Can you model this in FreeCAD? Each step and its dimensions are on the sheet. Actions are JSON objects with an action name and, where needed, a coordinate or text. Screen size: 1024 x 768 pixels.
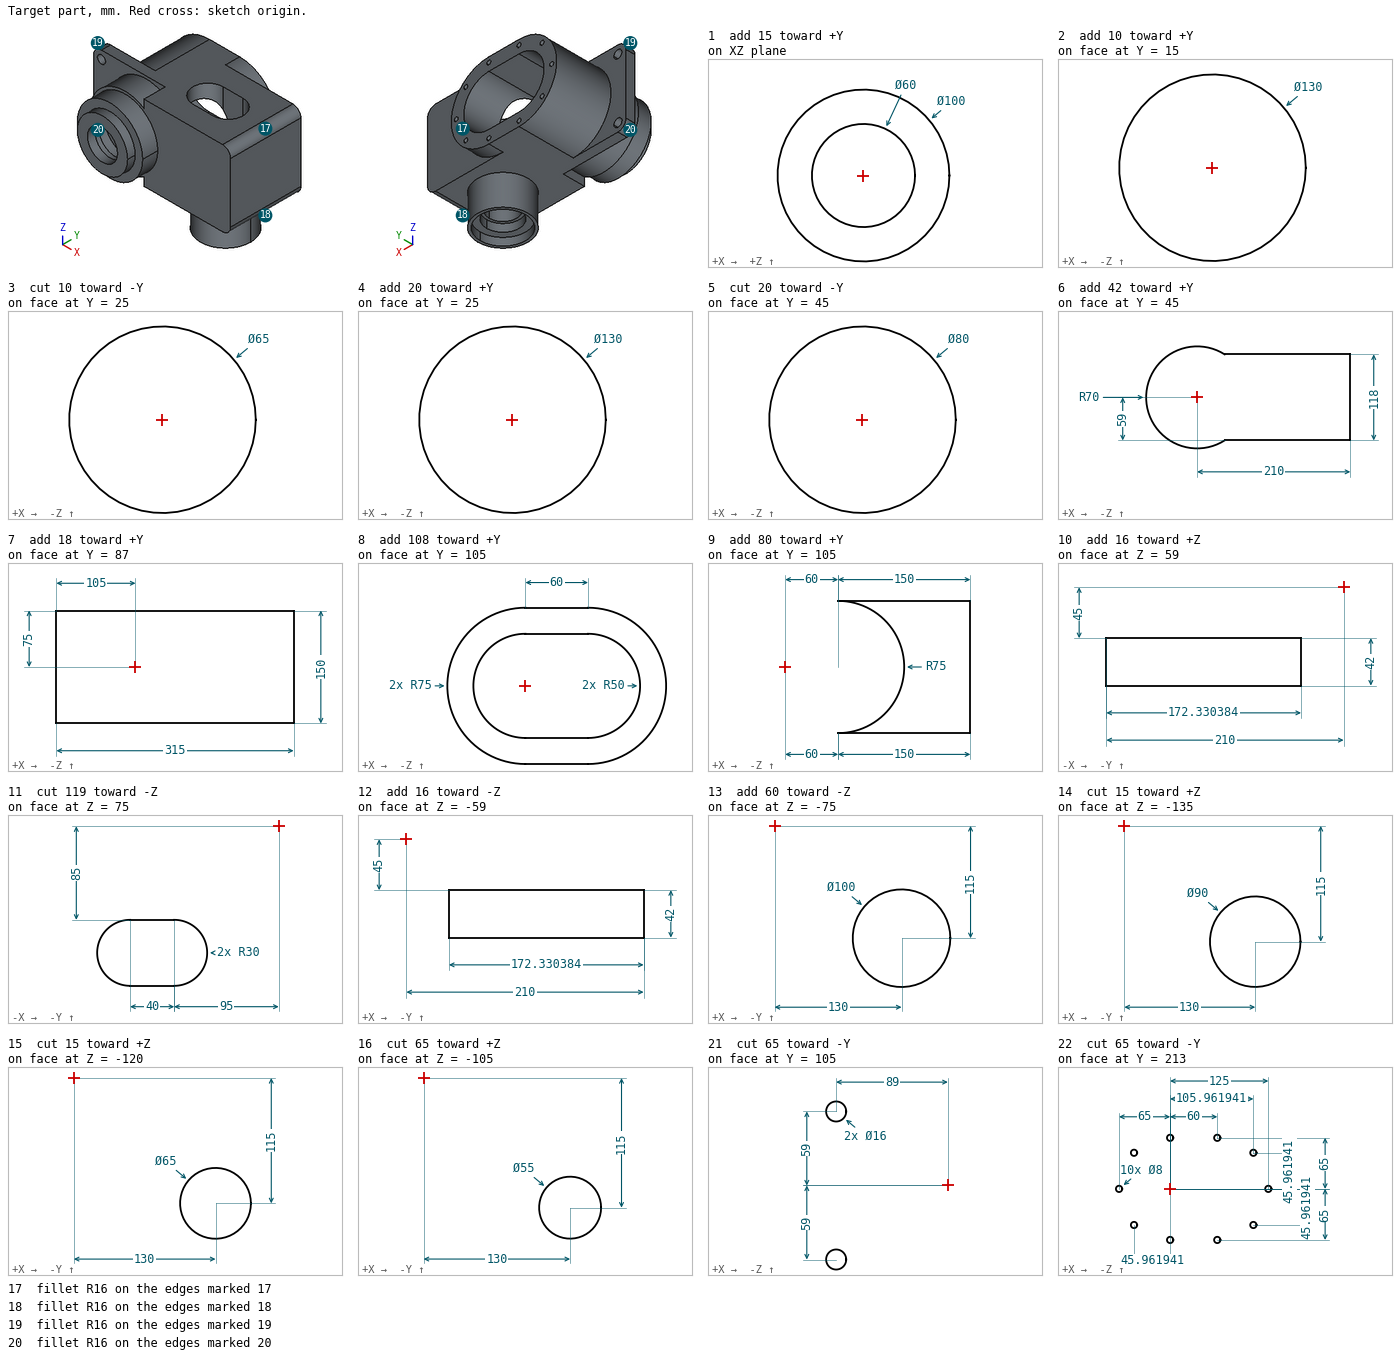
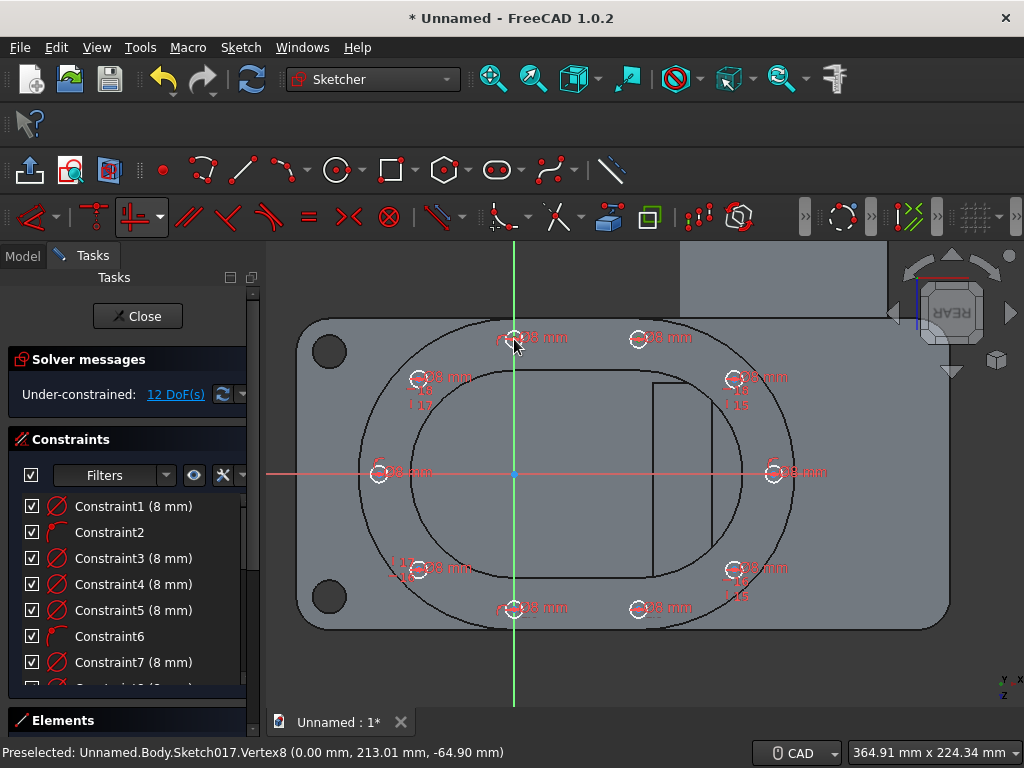
{"action": "key", "text": "h"}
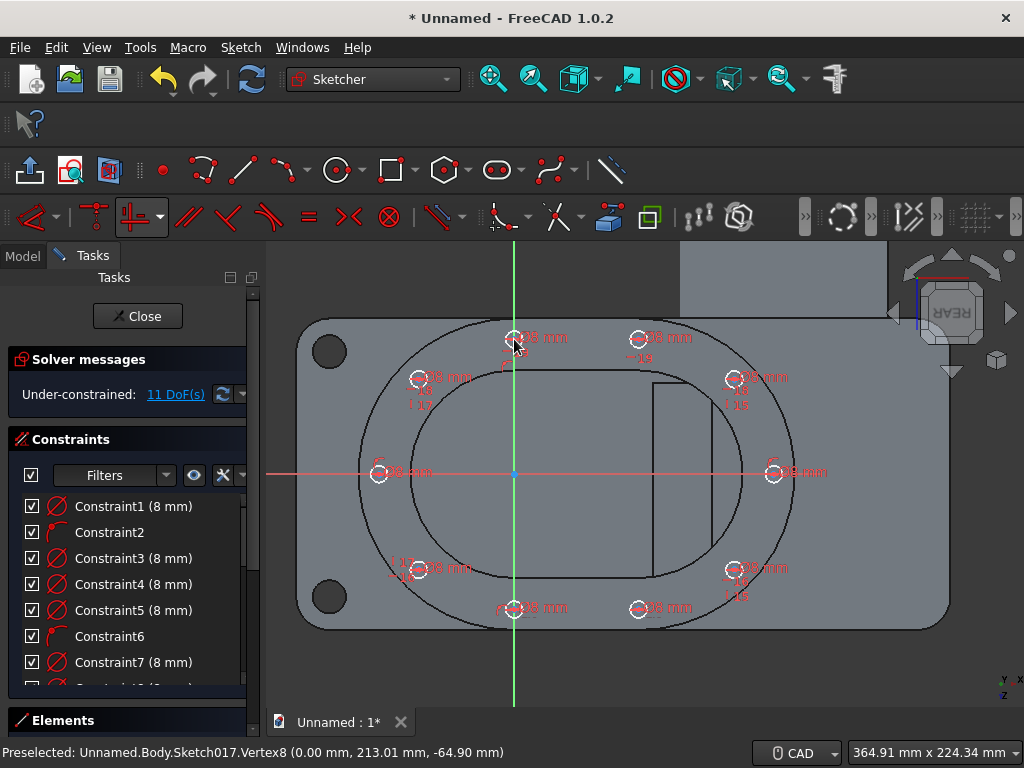
{"action": "left_click", "coordinate": [639, 339]}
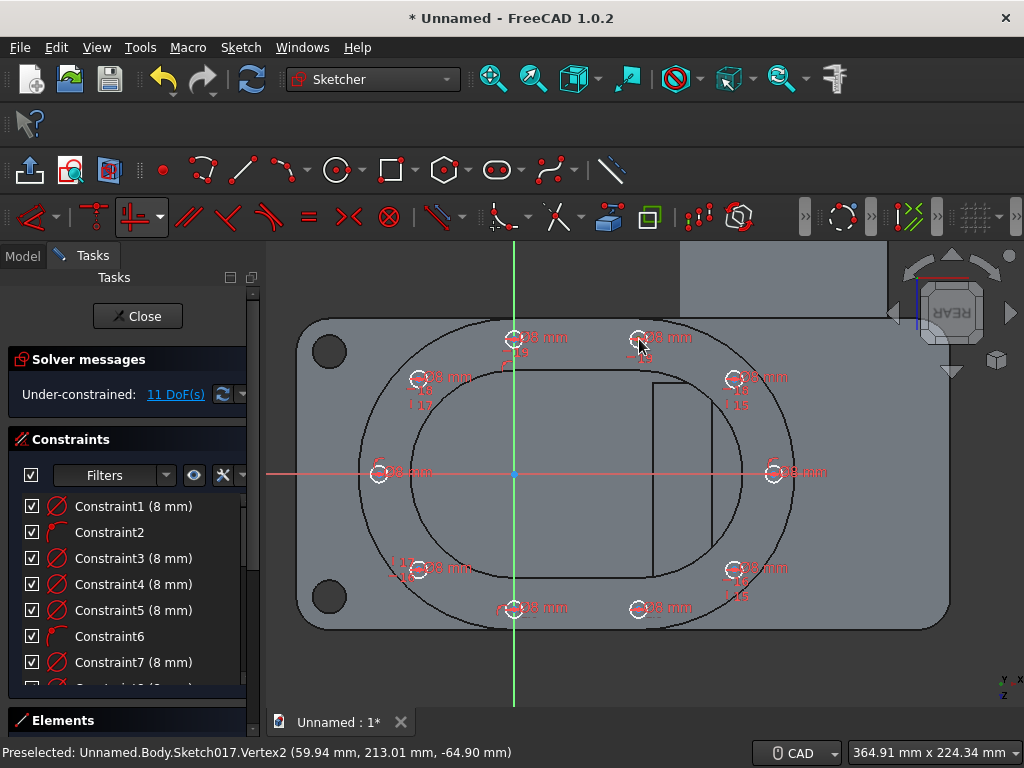
{"action": "left_click", "coordinate": [639, 610]}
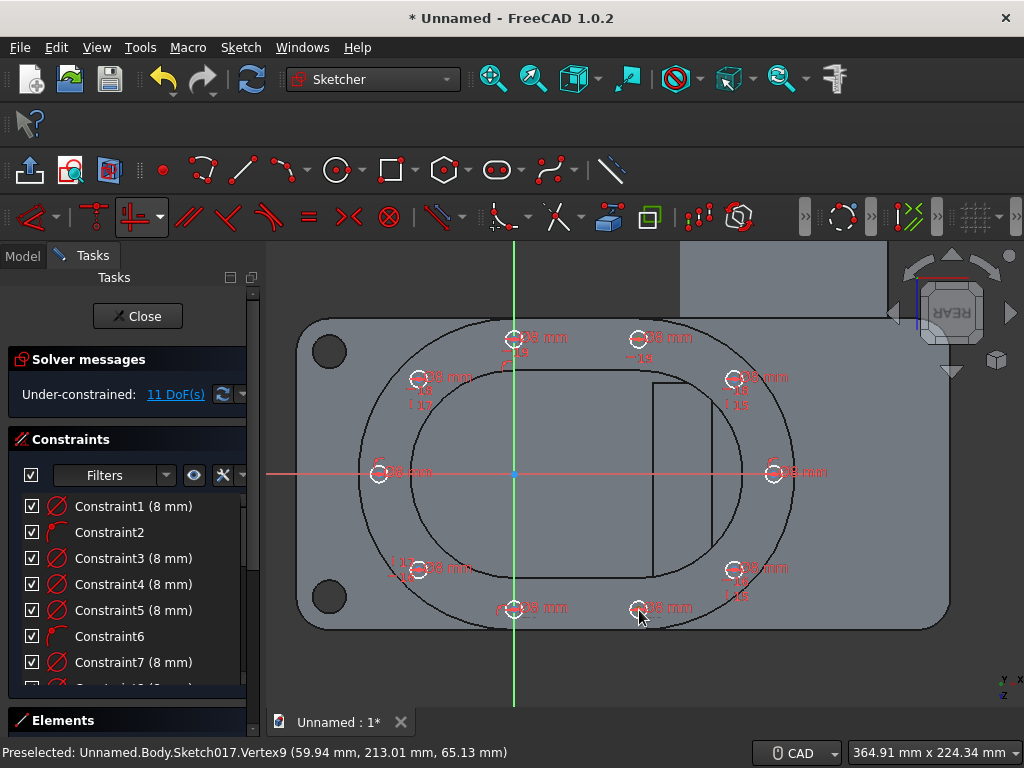
{"action": "key", "text": "v"}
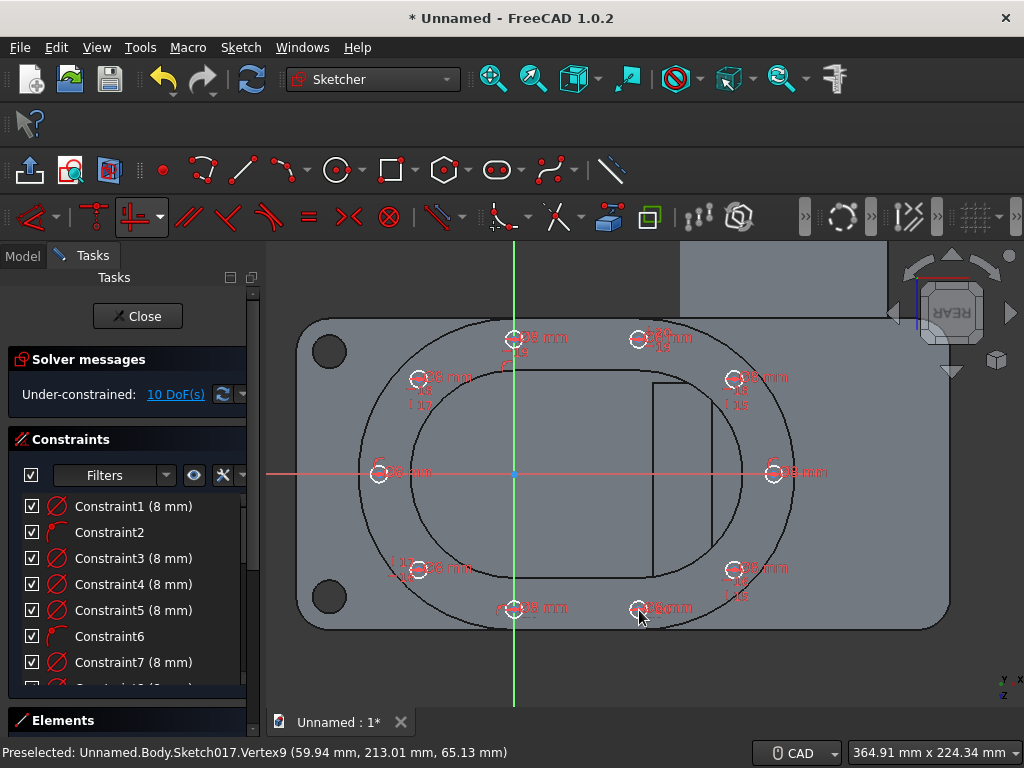
{"action": "left_click", "coordinate": [639, 610]}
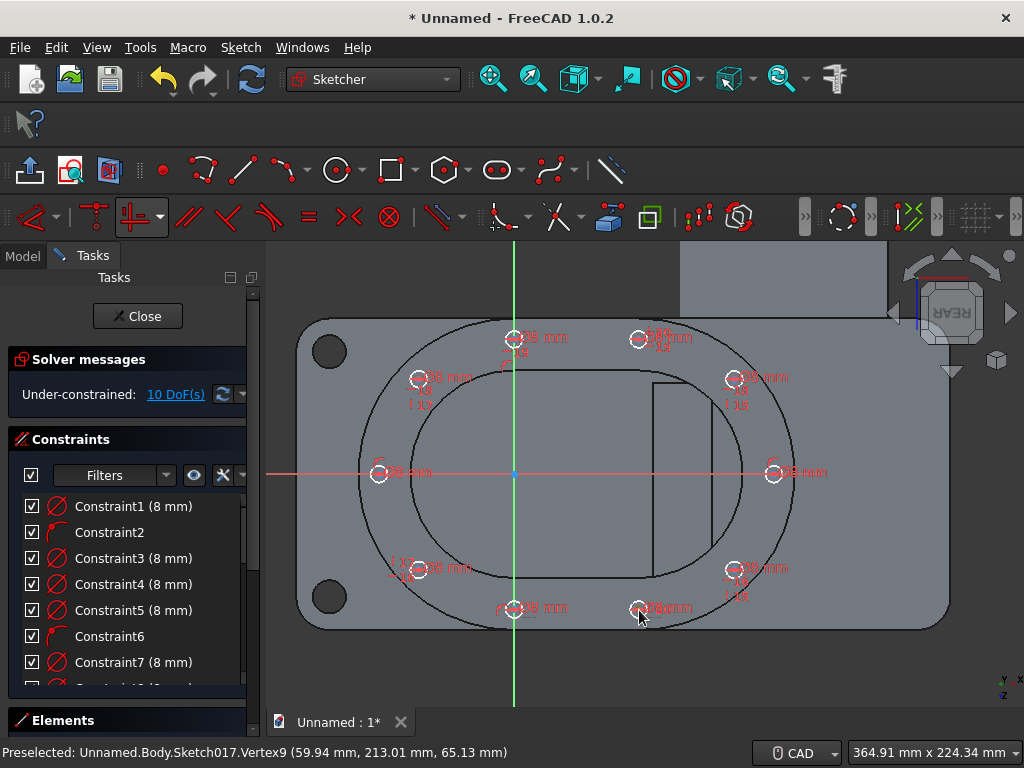
{"action": "left_click", "coordinate": [514, 610]}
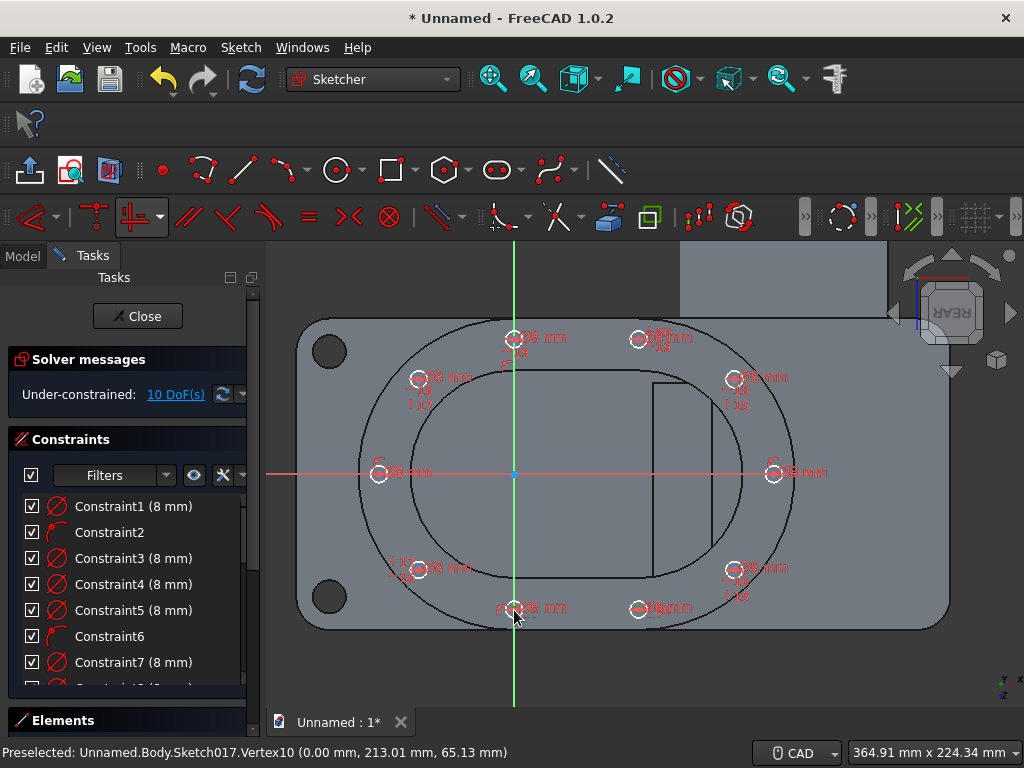
{"action": "left_click", "coordinate": [162, 218]}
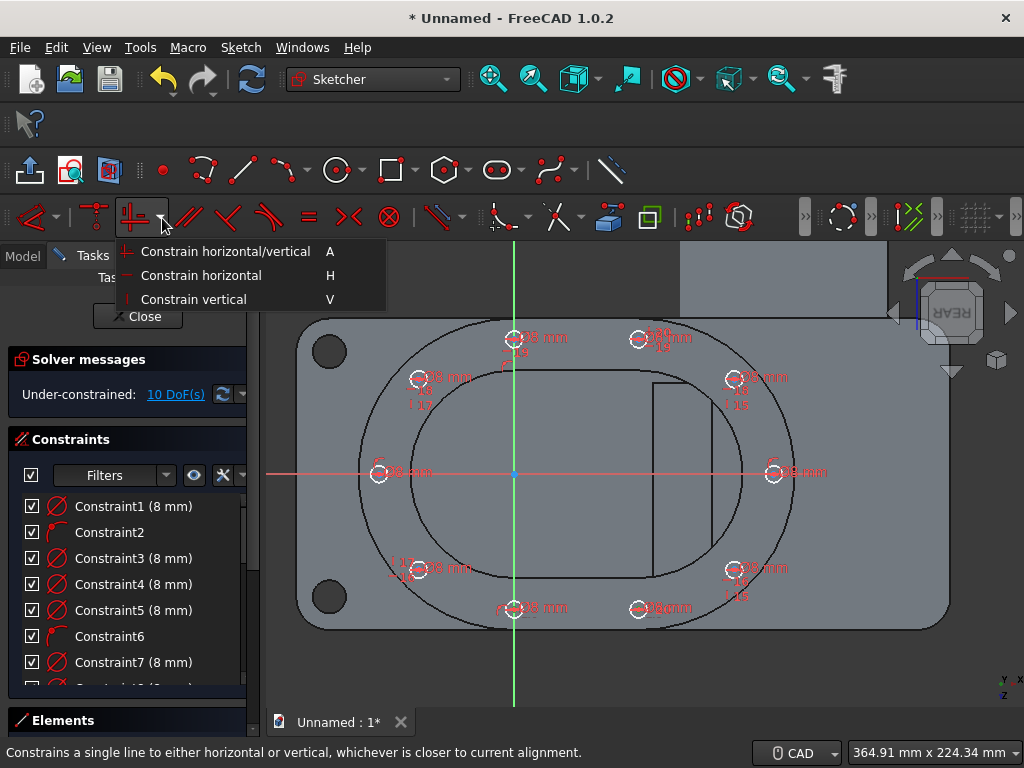
{"action": "left_click", "coordinate": [251, 275]}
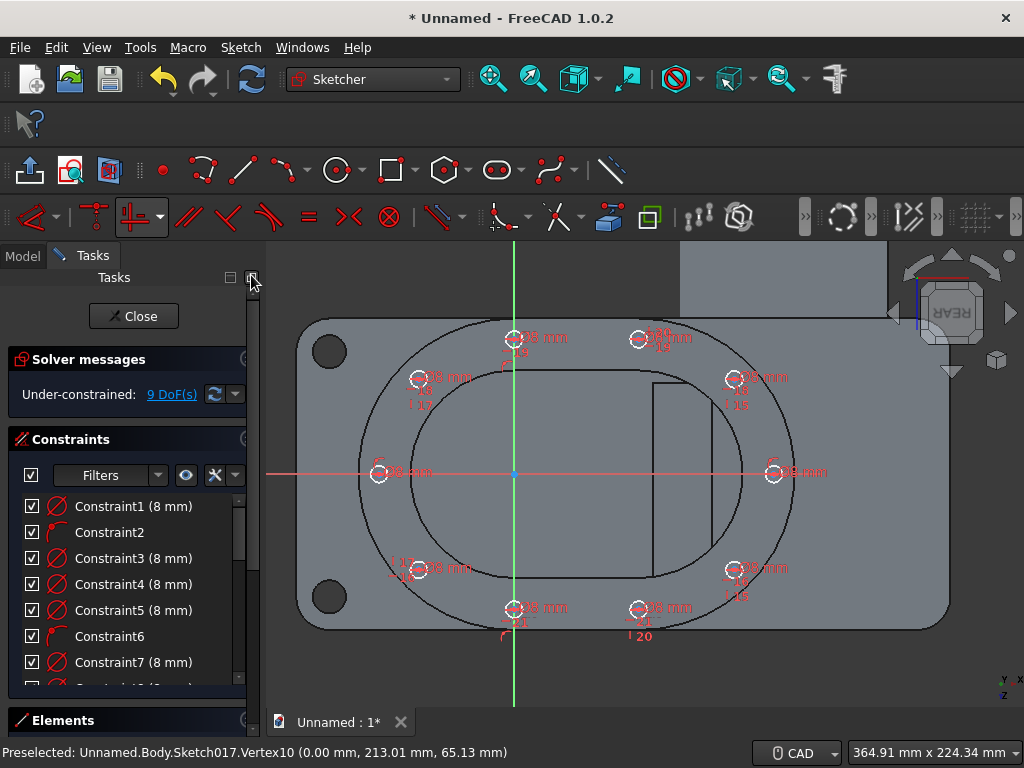
{"action": "left_click", "coordinate": [32, 218]}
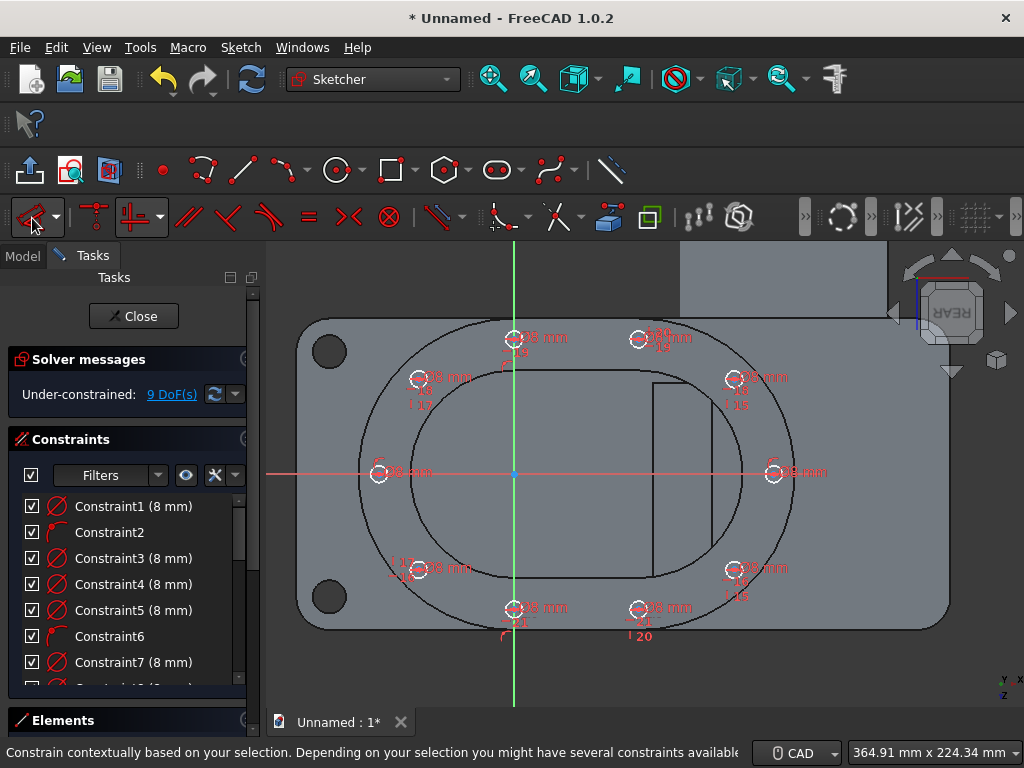
{"action": "left_click", "coordinate": [379, 474]}
{"action": "left_click", "coordinate": [447, 508]}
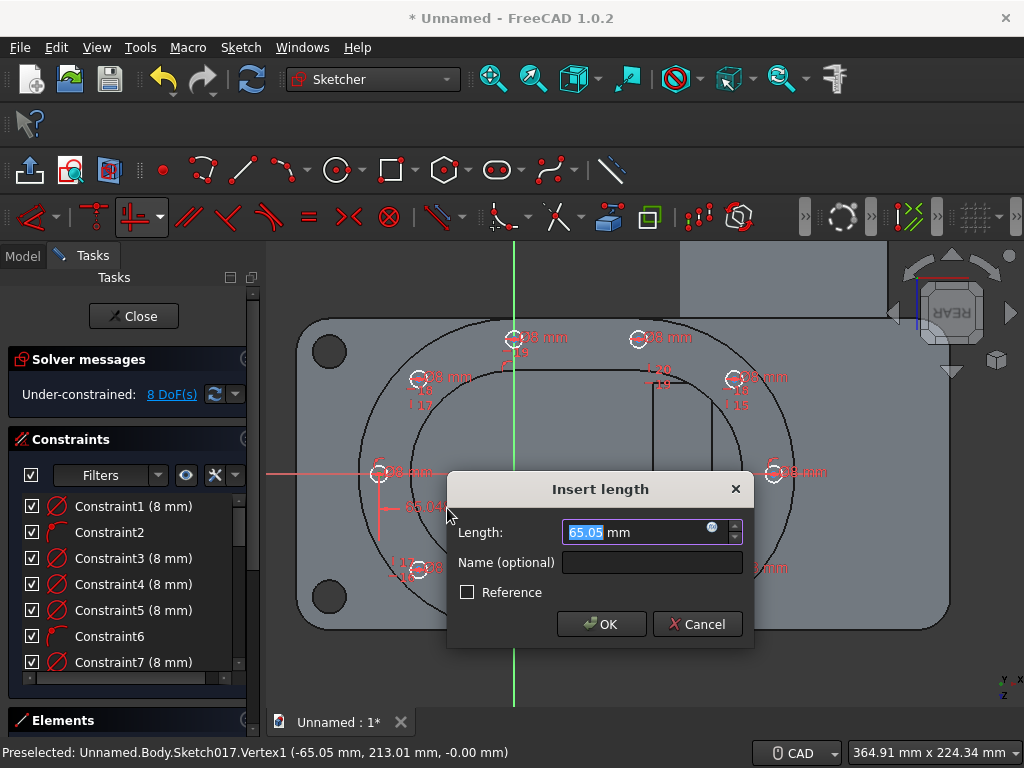
{"action": "type", "text": "65"}
{"action": "key", "text": "Return"}